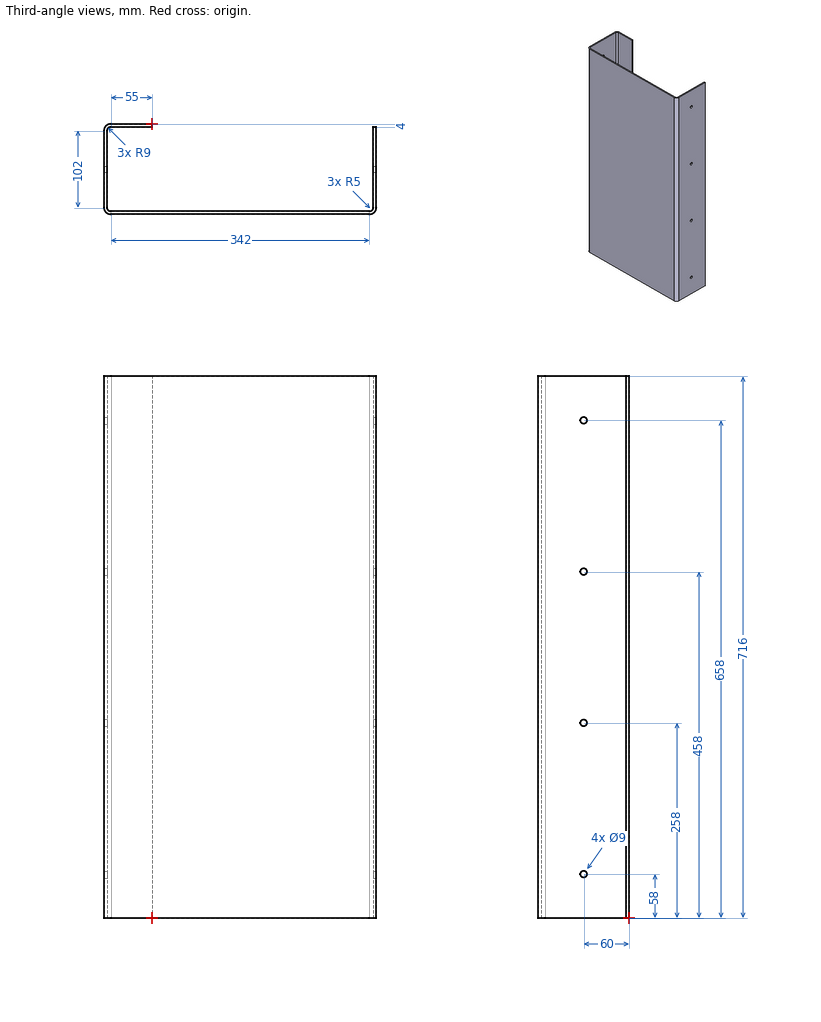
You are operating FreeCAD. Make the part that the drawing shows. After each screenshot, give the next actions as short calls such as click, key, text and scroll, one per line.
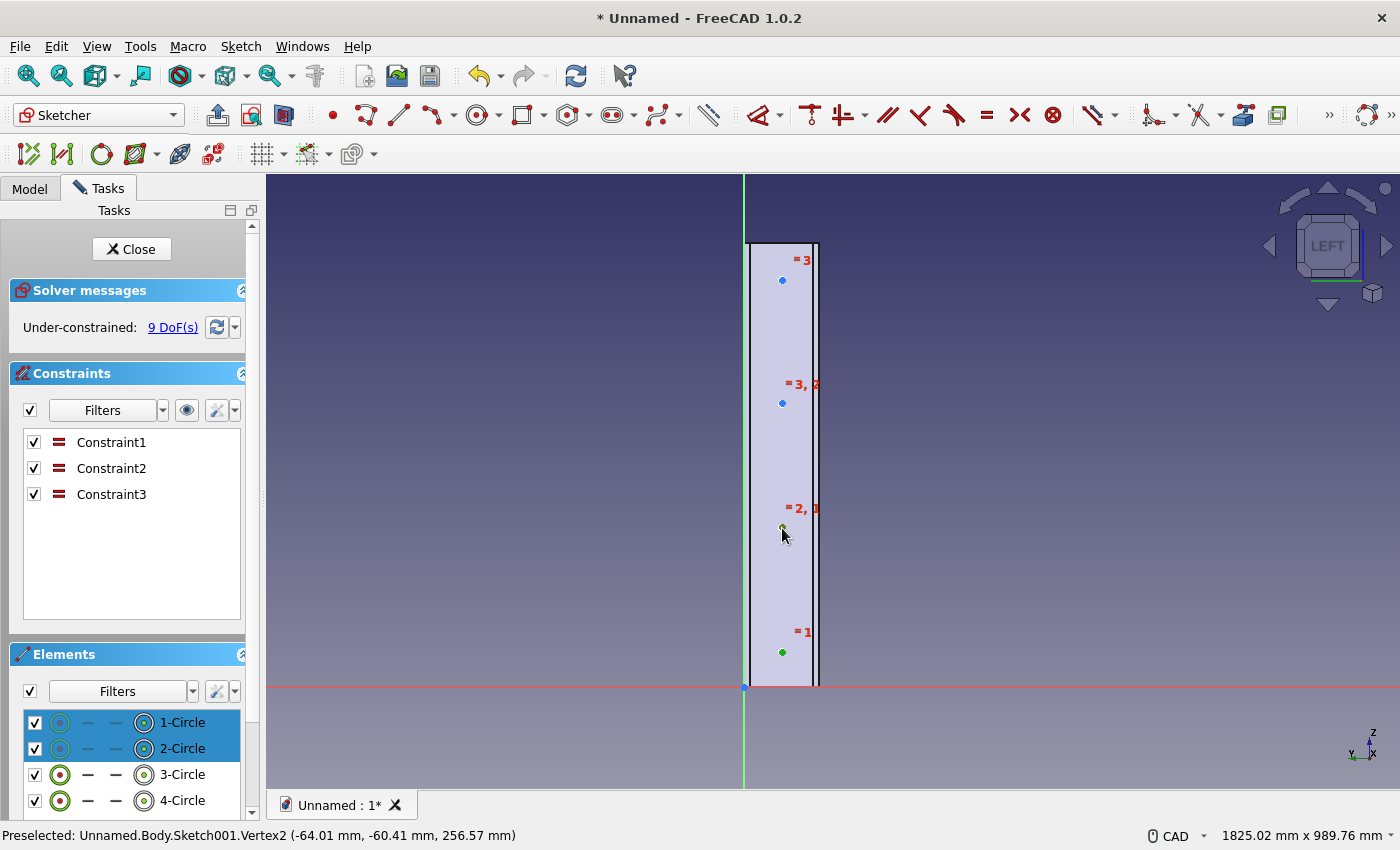
click(864, 116)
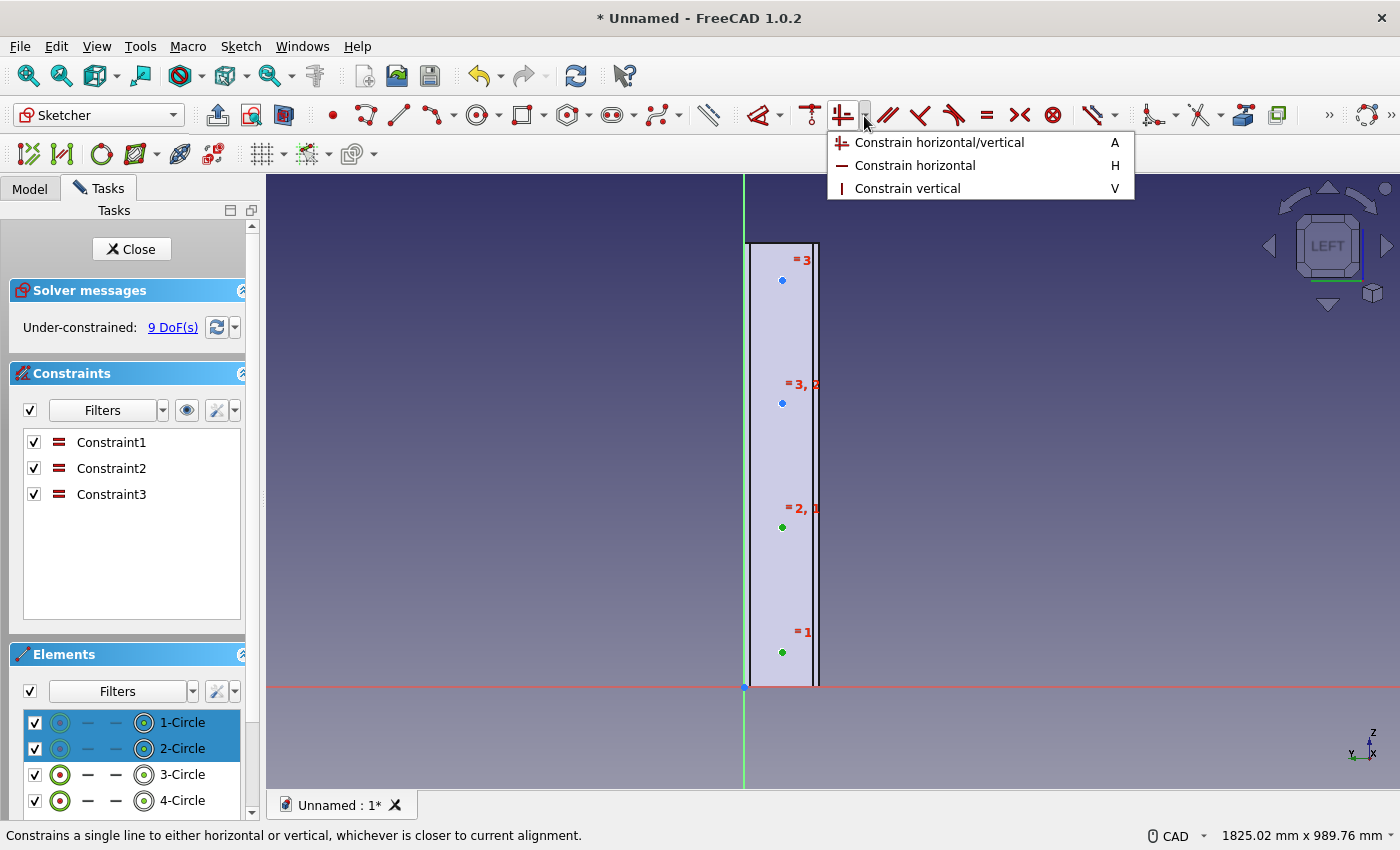
click(981, 188)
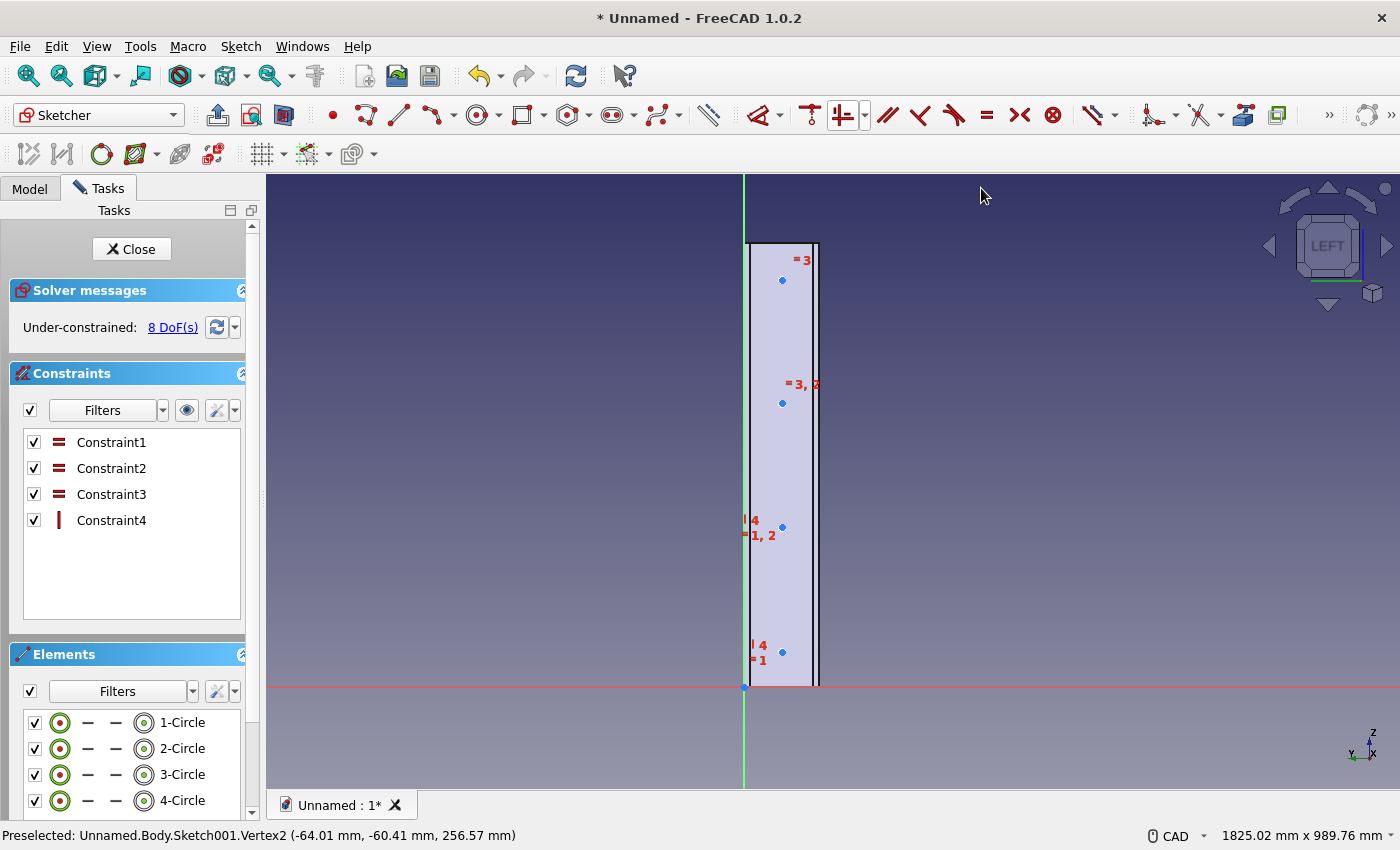
click(782, 528)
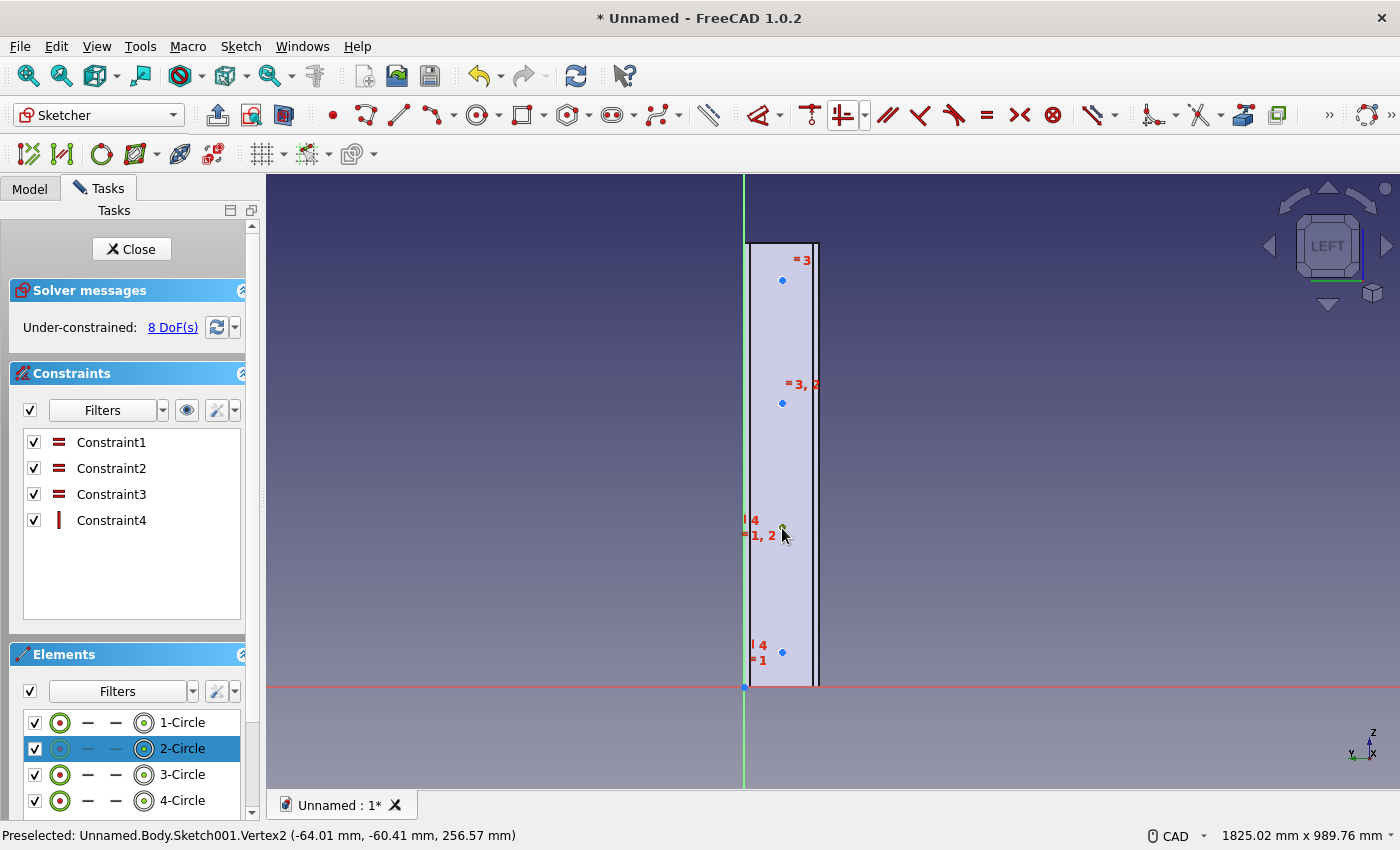
click(782, 404)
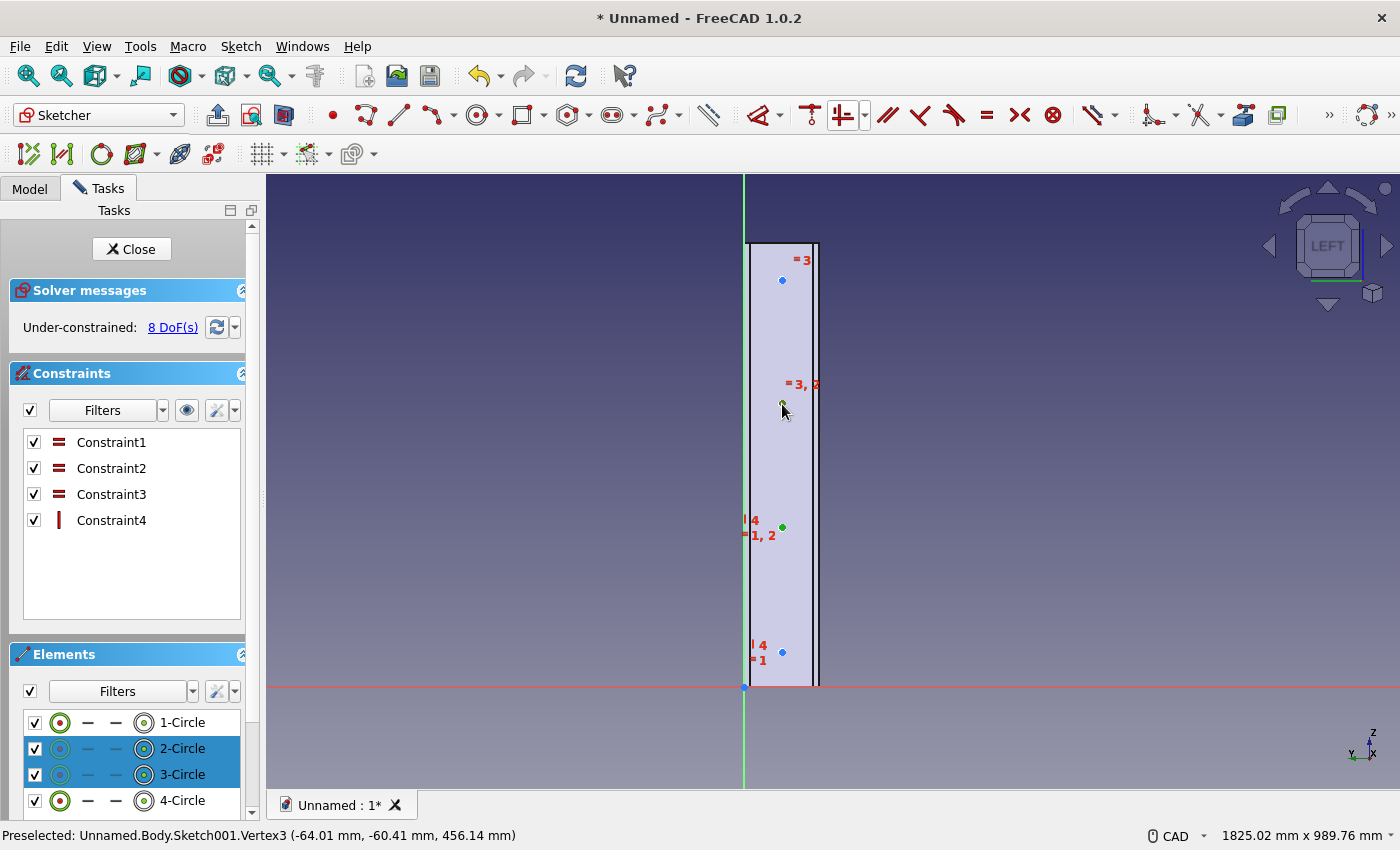
click(864, 116)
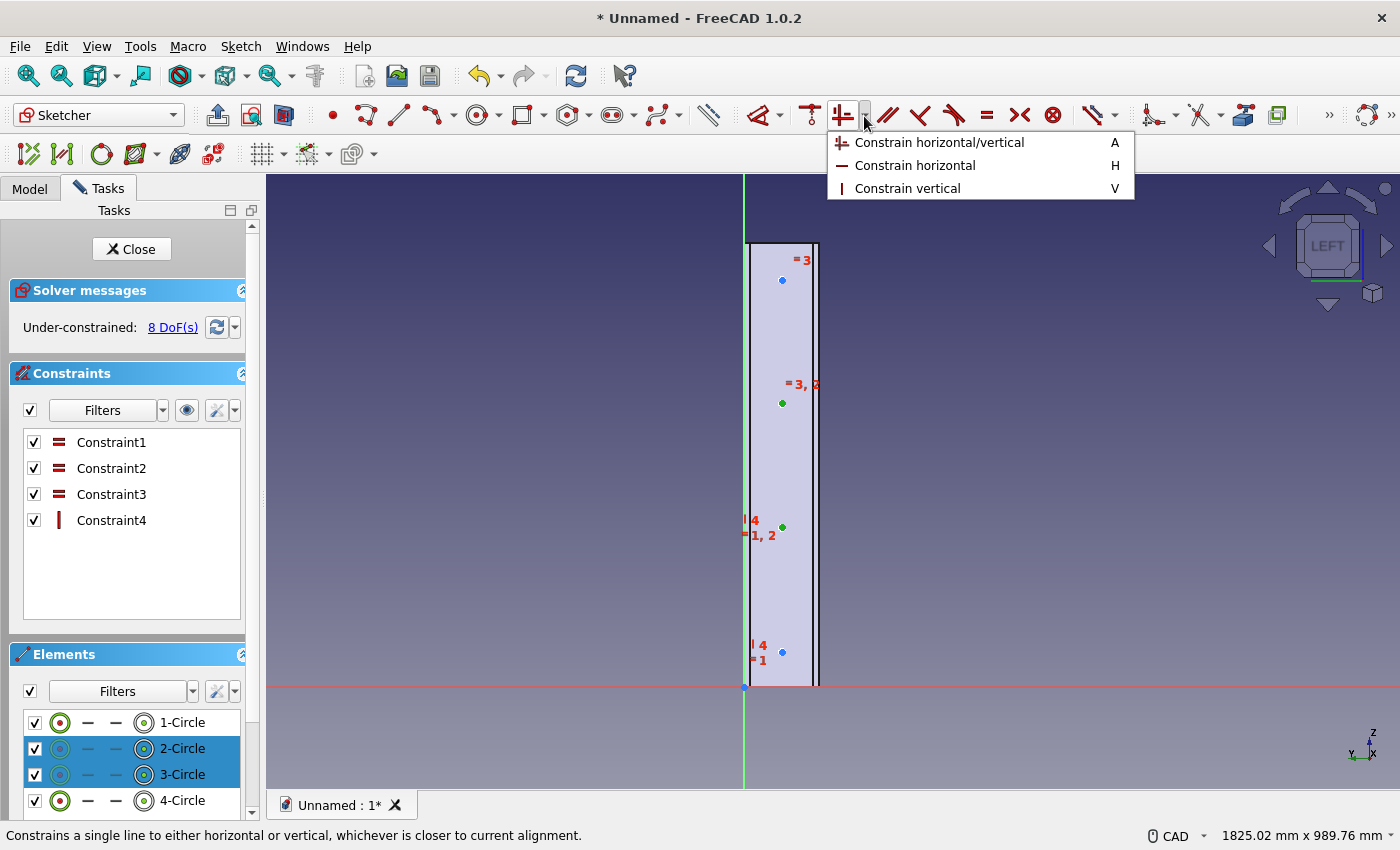
click(981, 188)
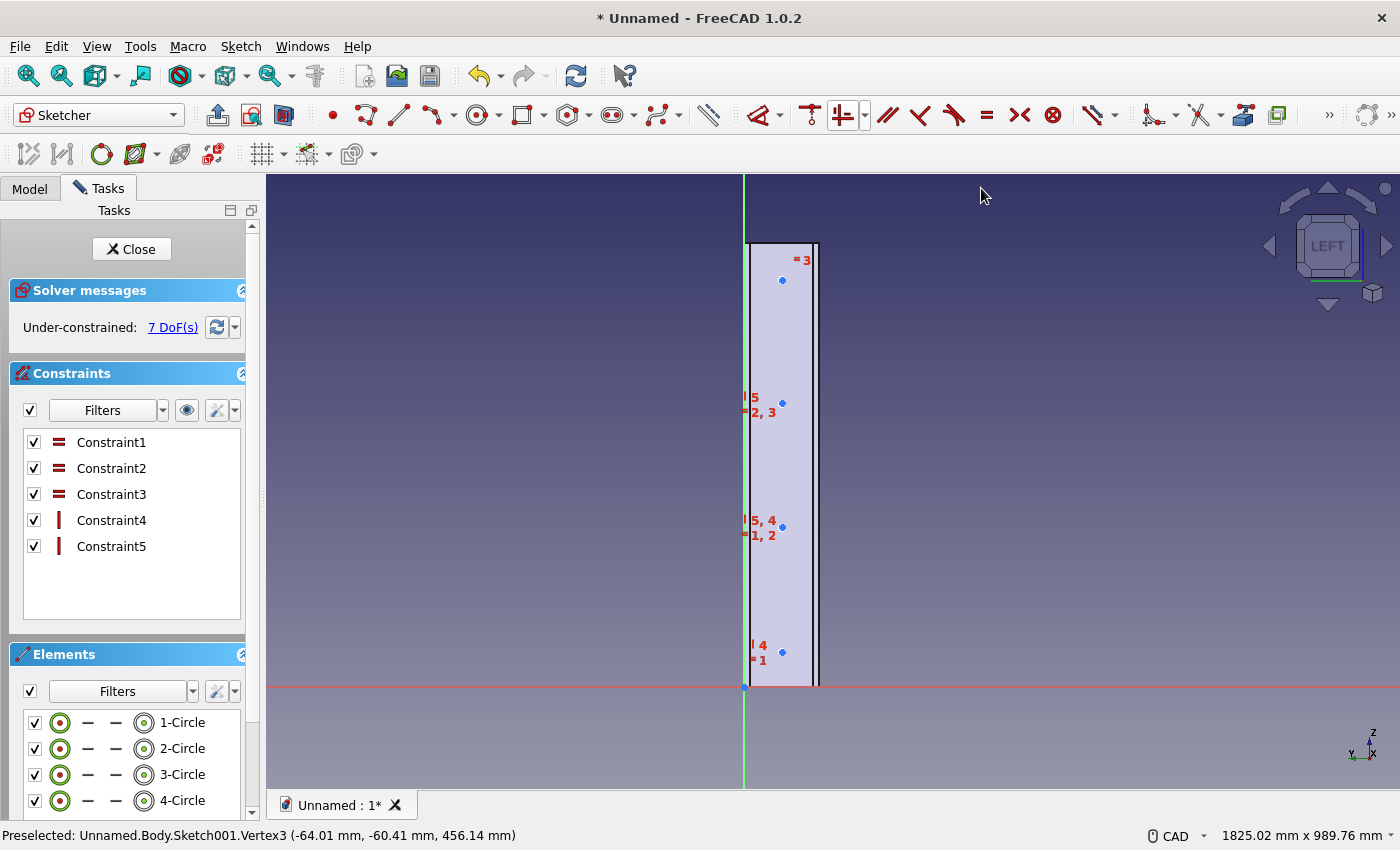
click(782, 404)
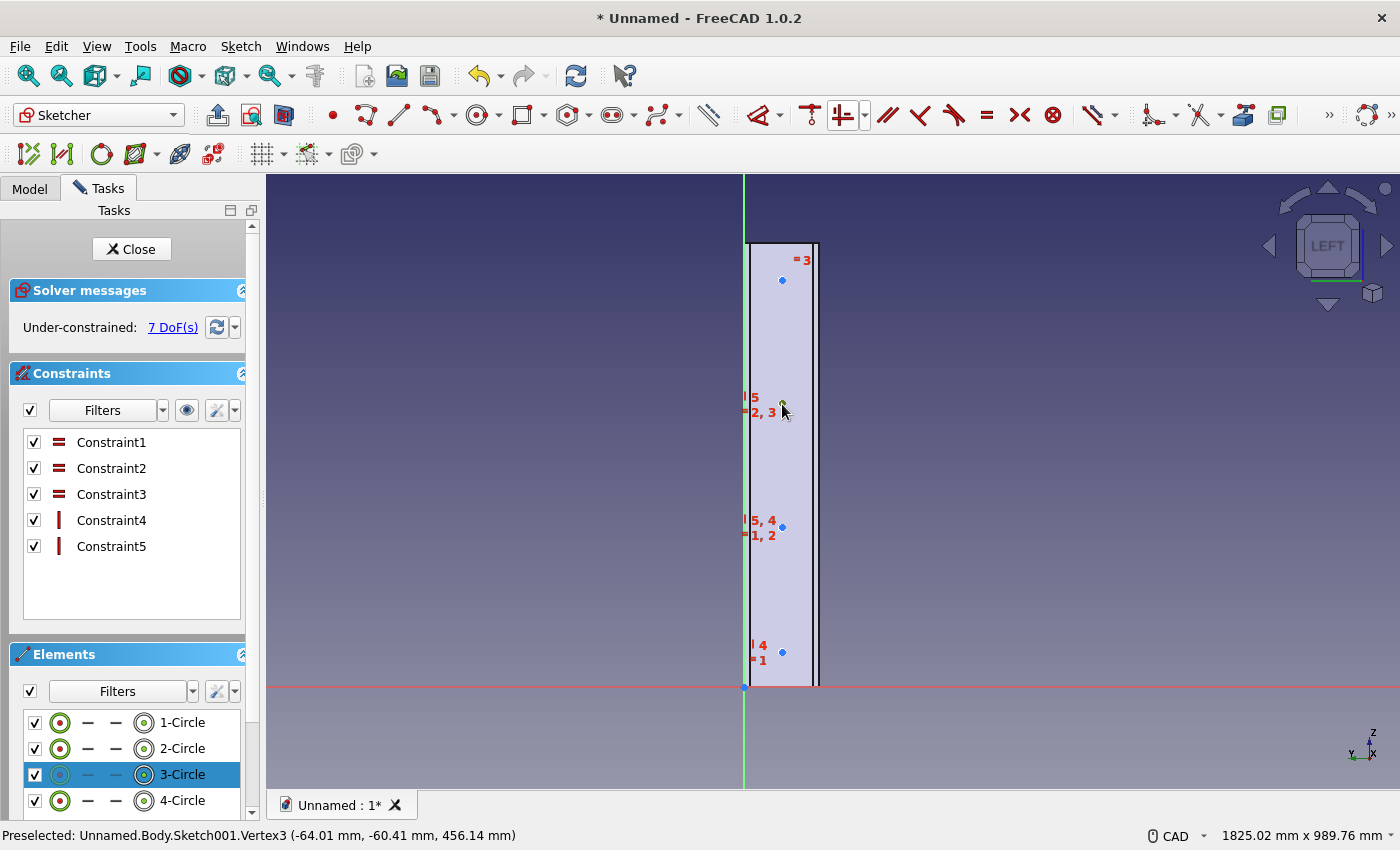
click(782, 280)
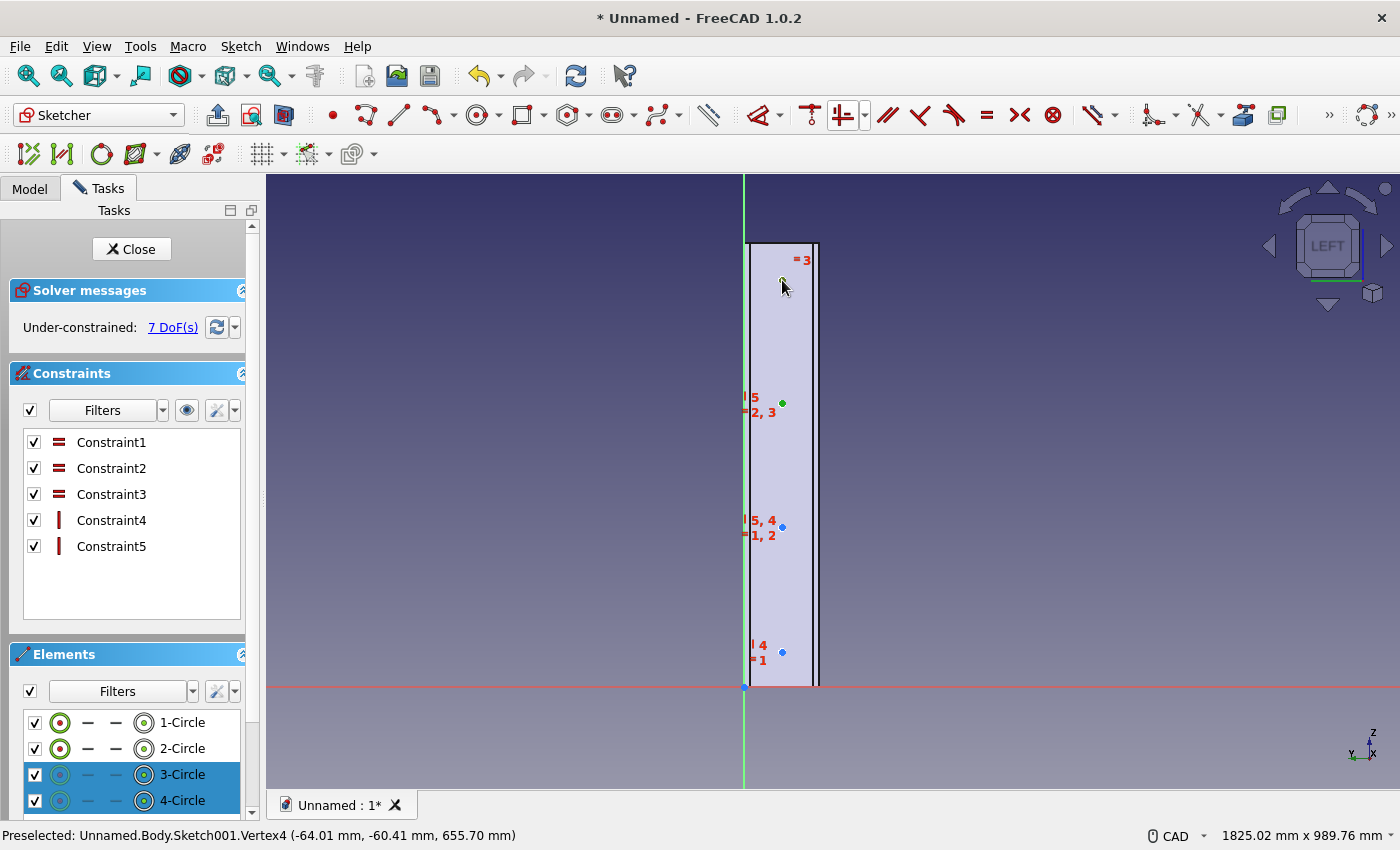
click(864, 116)